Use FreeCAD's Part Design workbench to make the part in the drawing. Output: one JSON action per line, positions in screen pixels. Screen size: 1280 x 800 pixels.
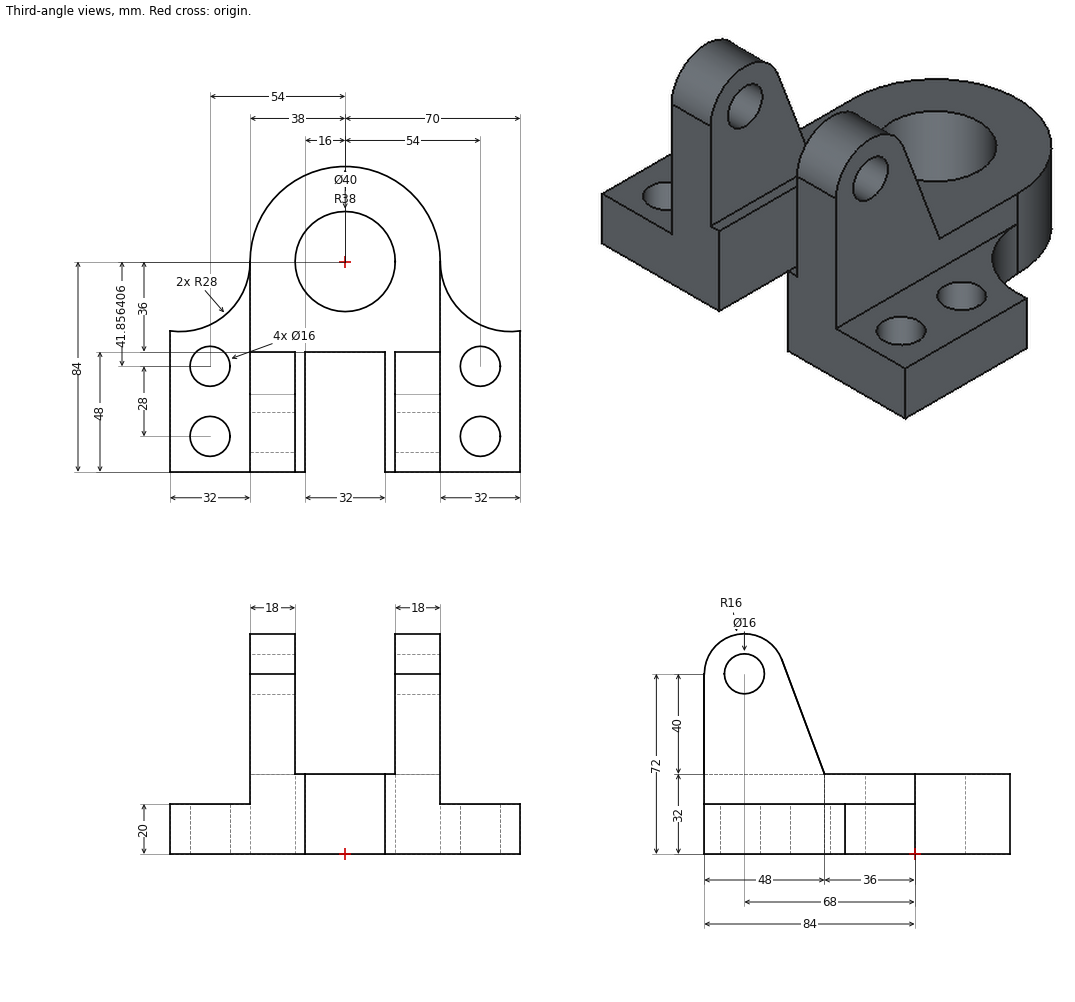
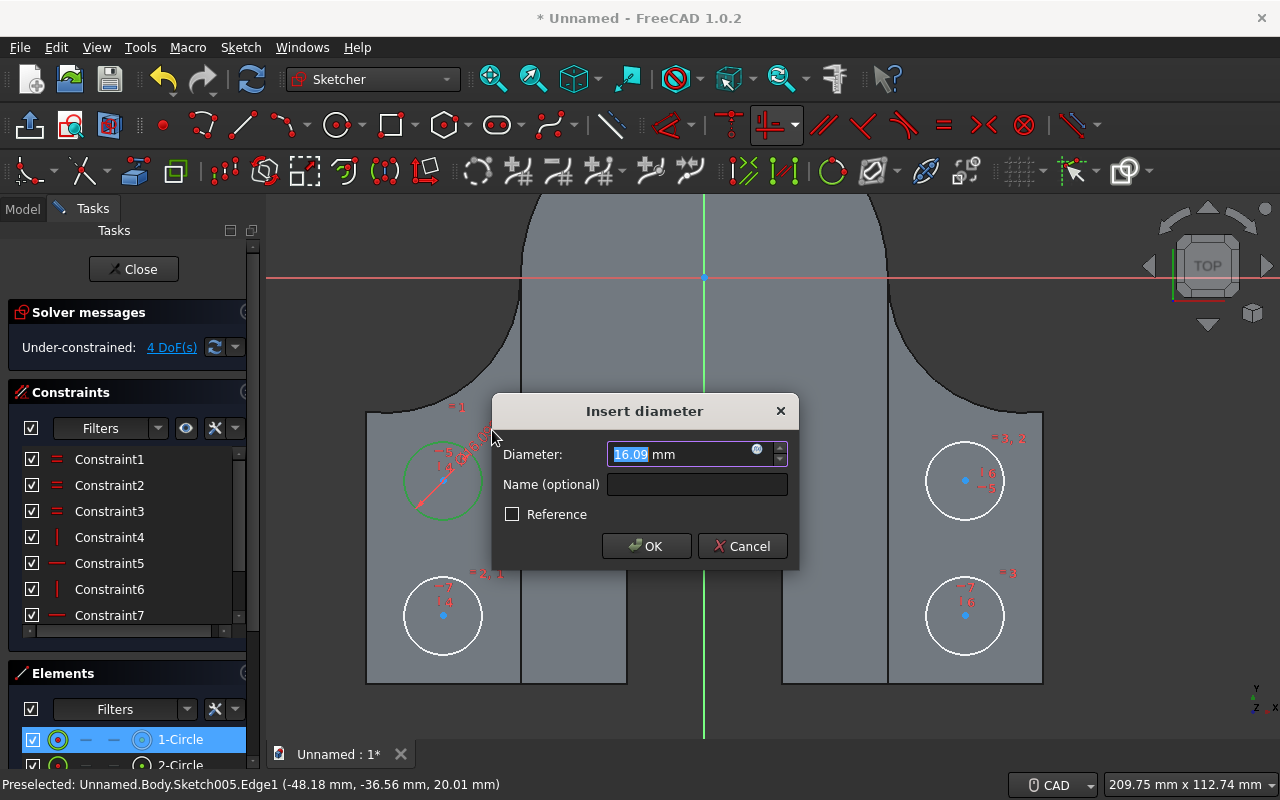
{"action": "type", "text": "16"}
{"action": "key", "text": "Return"}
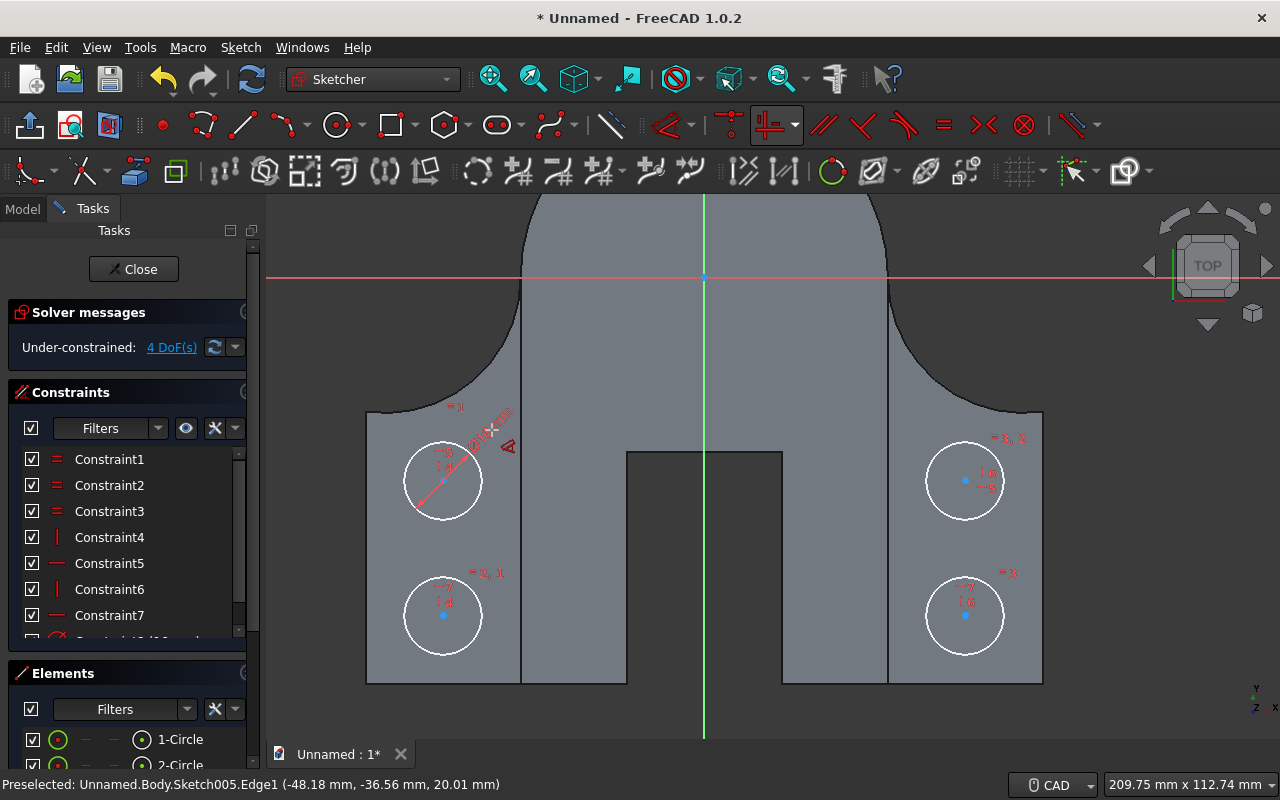
{"action": "left_click", "coordinate": [443, 481]}
{"action": "left_click", "coordinate": [574, 244]}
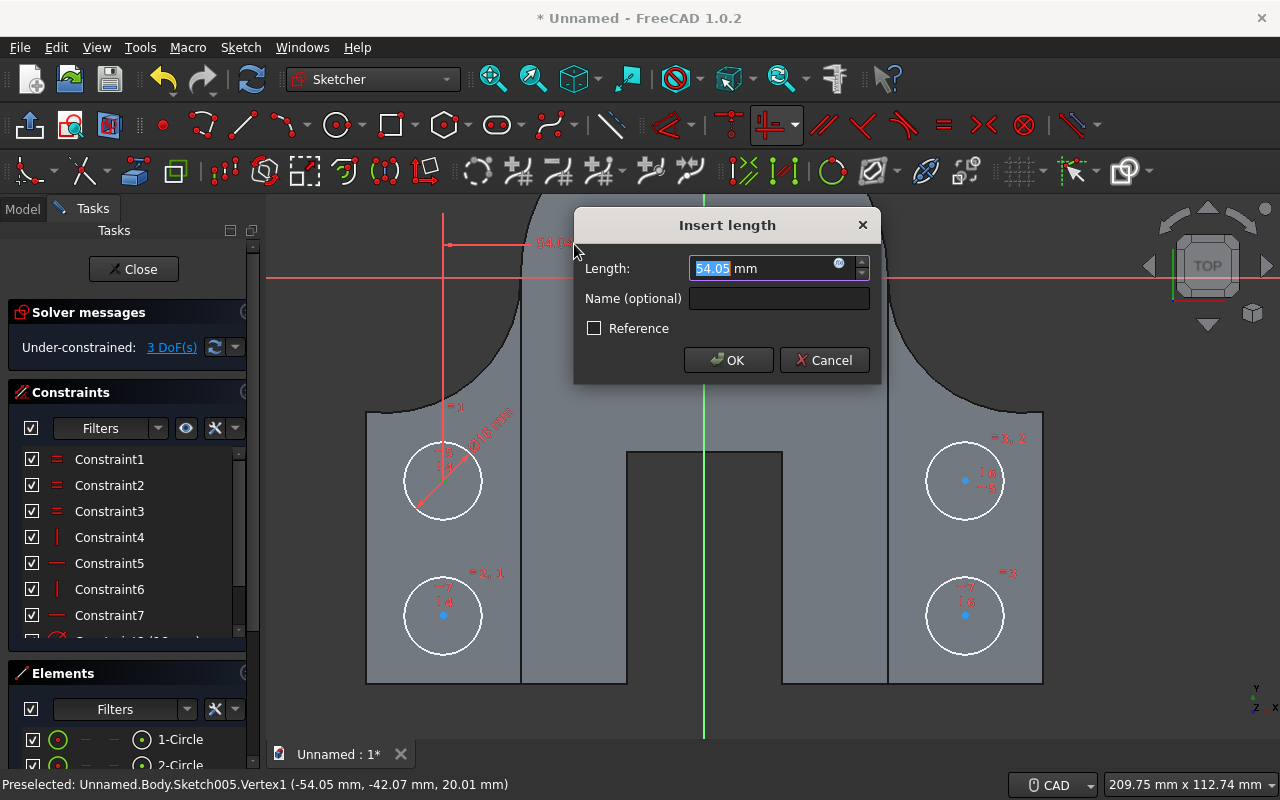
{"action": "type", "text": "54"}
{"action": "key", "text": "Return"}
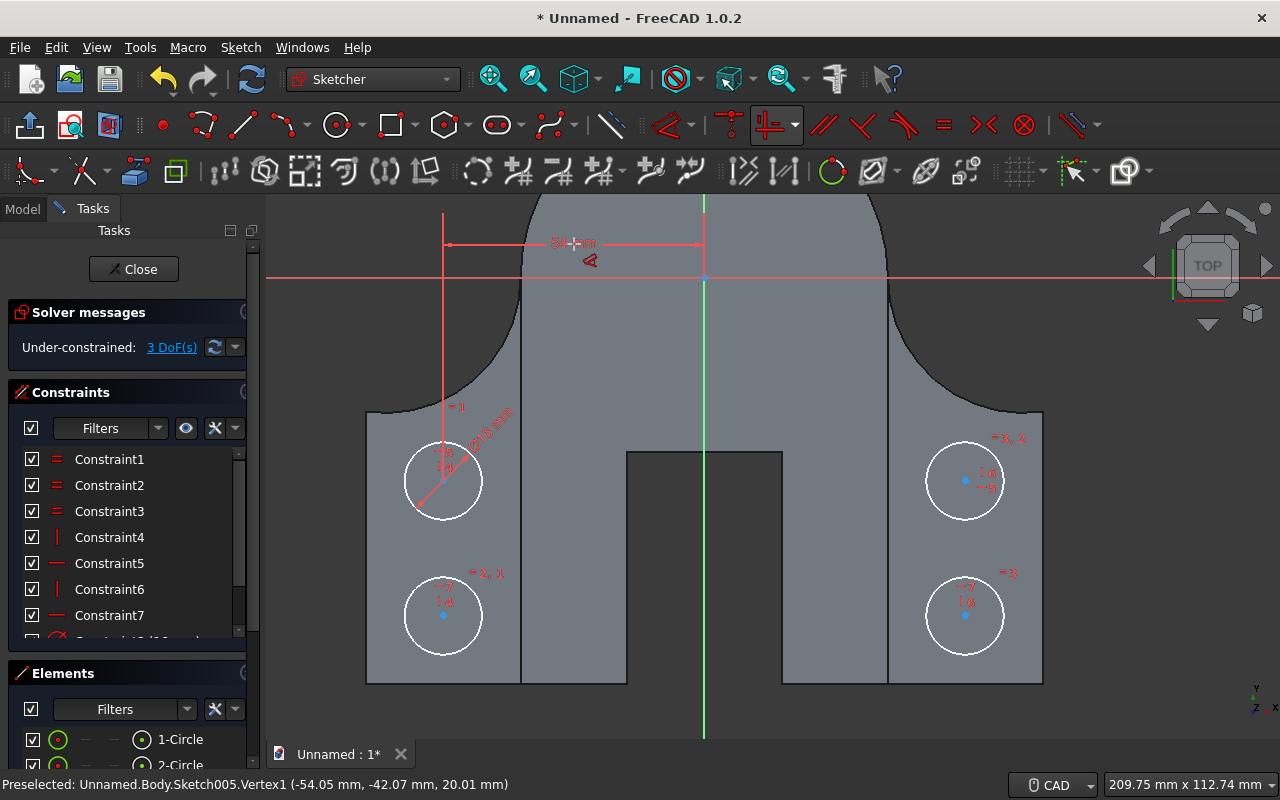
{"action": "left_click", "coordinate": [965, 481]}
{"action": "left_click", "coordinate": [835, 244]}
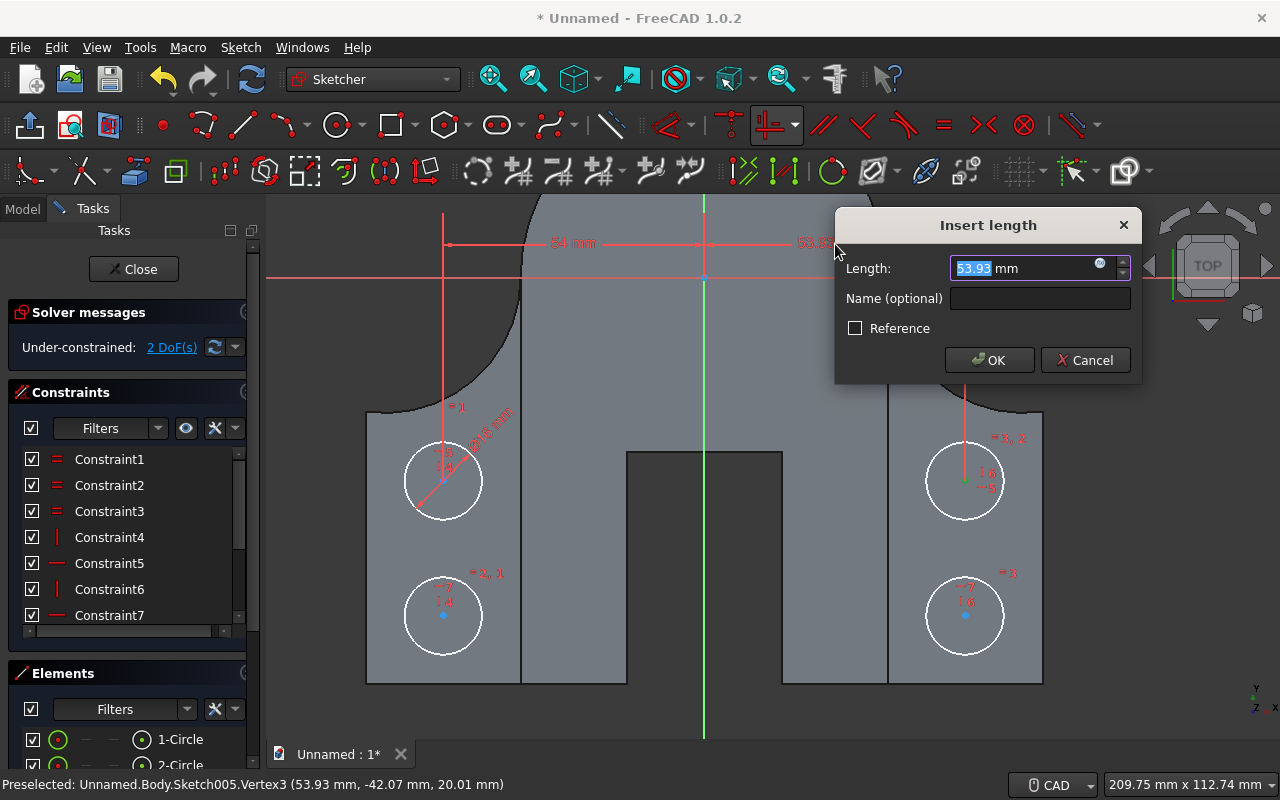
{"action": "type", "text": "54"}
{"action": "key", "text": "Return"}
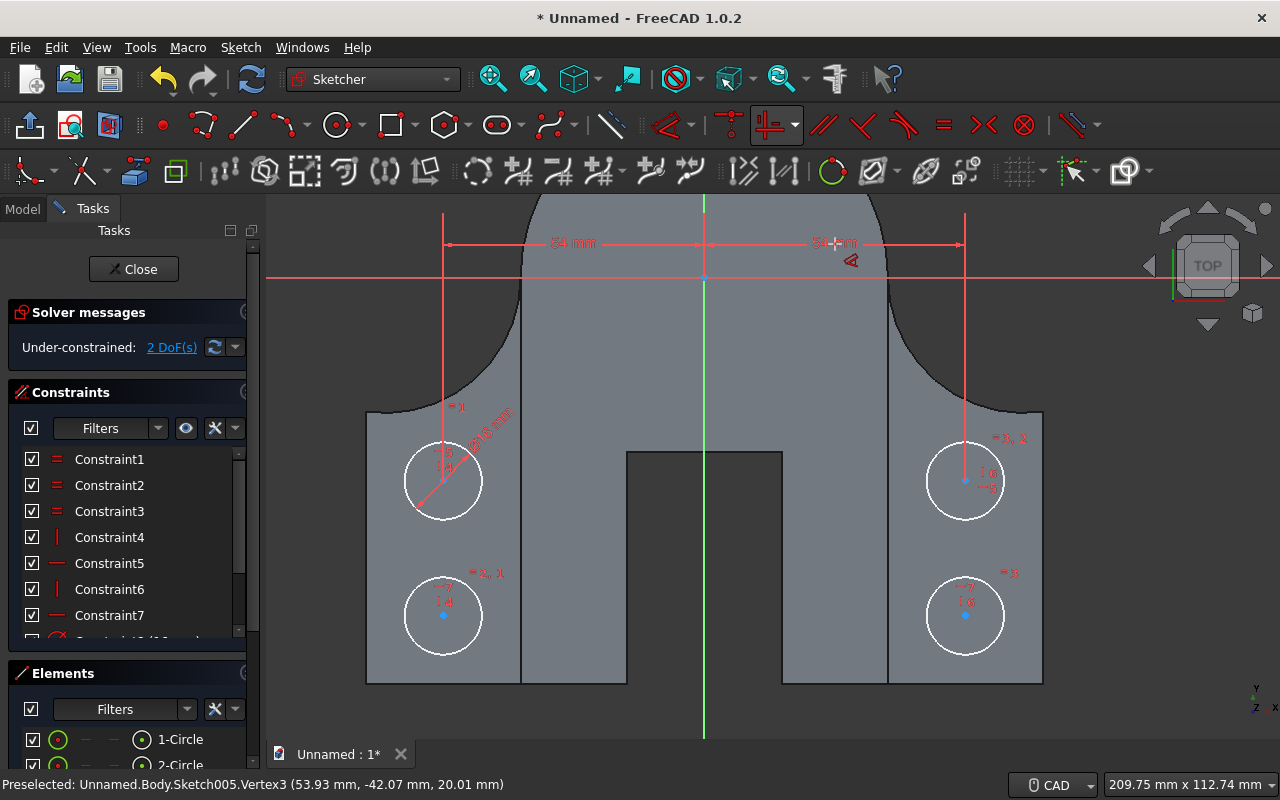
{"action": "left_click", "coordinate": [443, 481]}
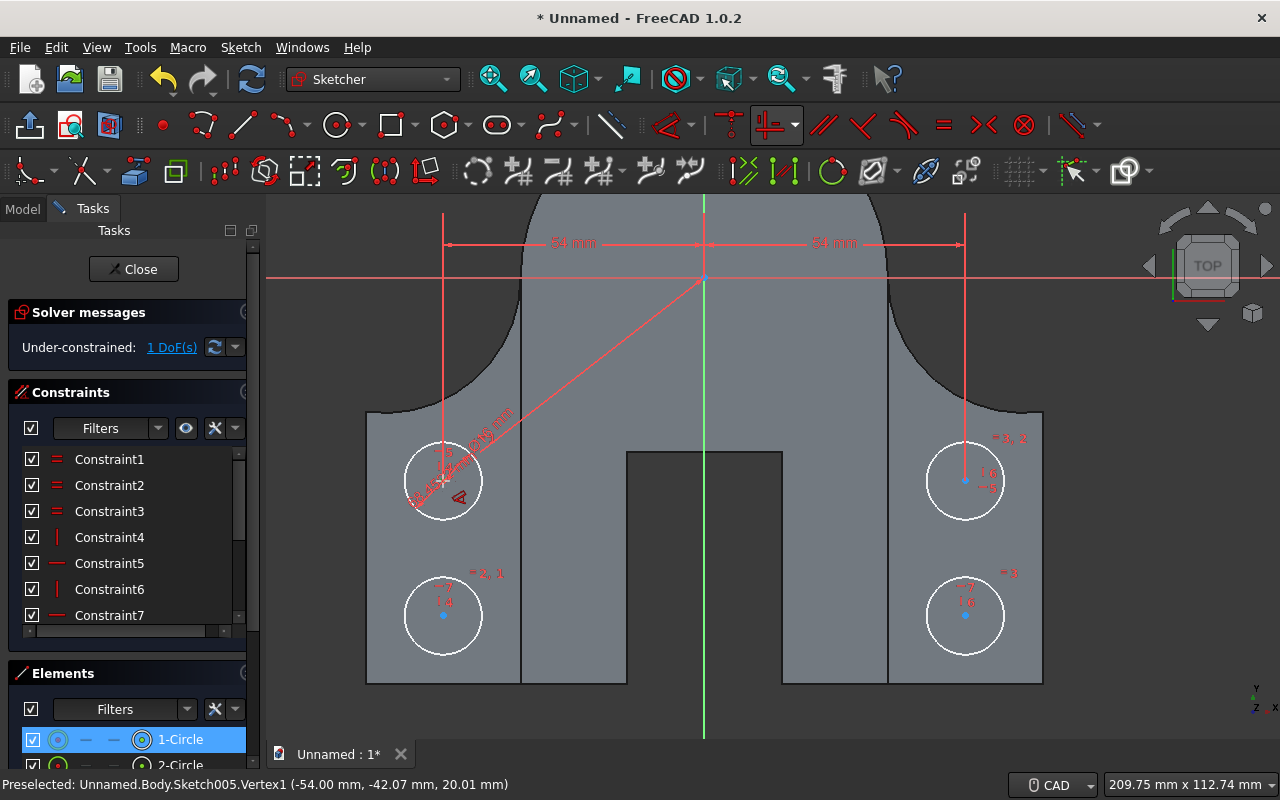
{"action": "left_click", "coordinate": [443, 616]}
{"action": "left_click", "coordinate": [409, 549]}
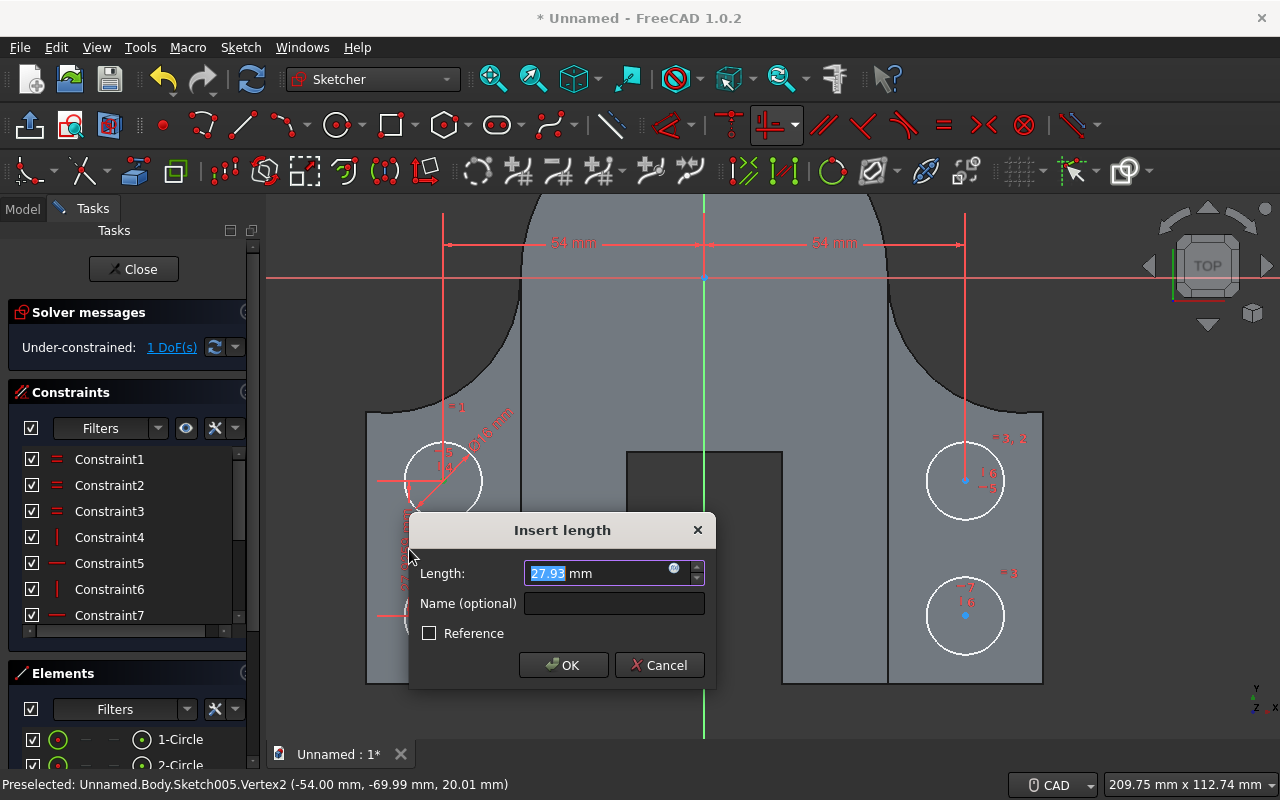
{"action": "type", "text": "28"}
{"action": "key", "text": "Return"}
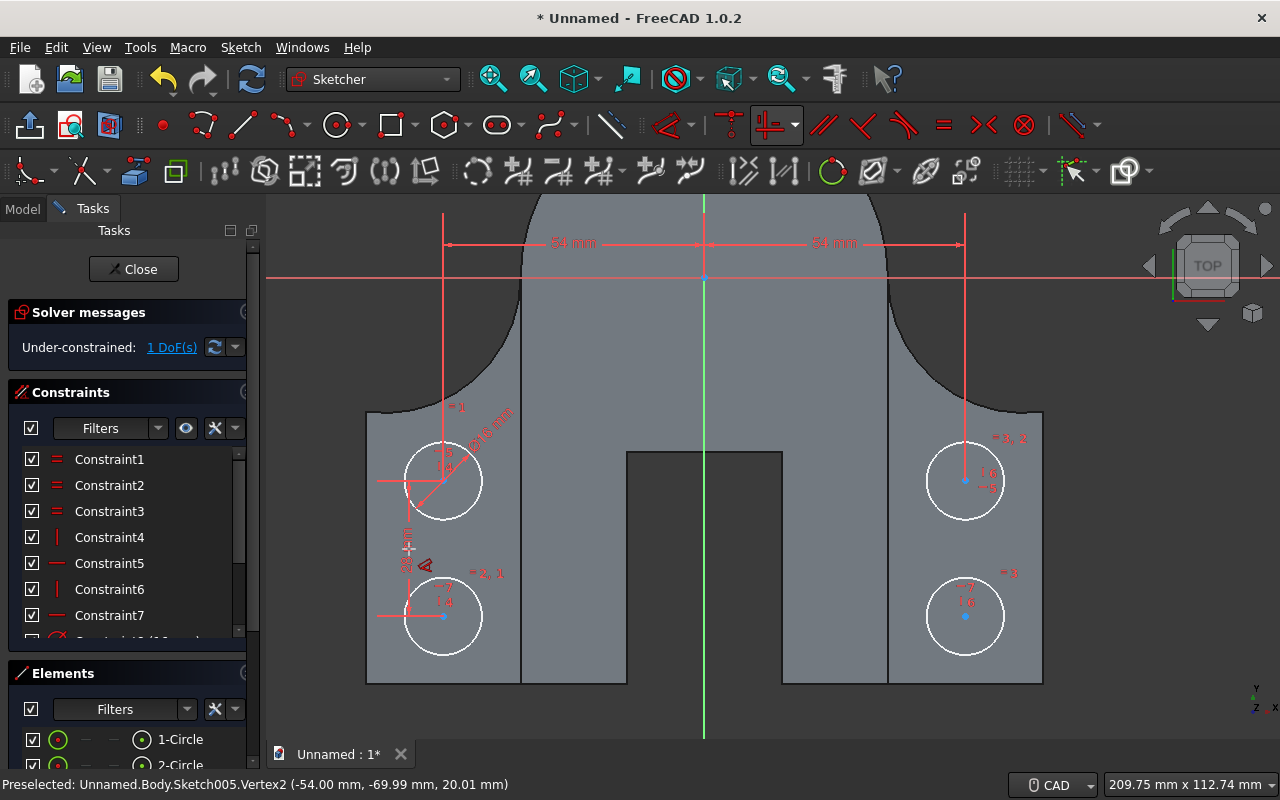
{"action": "left_click", "coordinate": [443, 481]}
{"action": "left_click", "coordinate": [409, 379]}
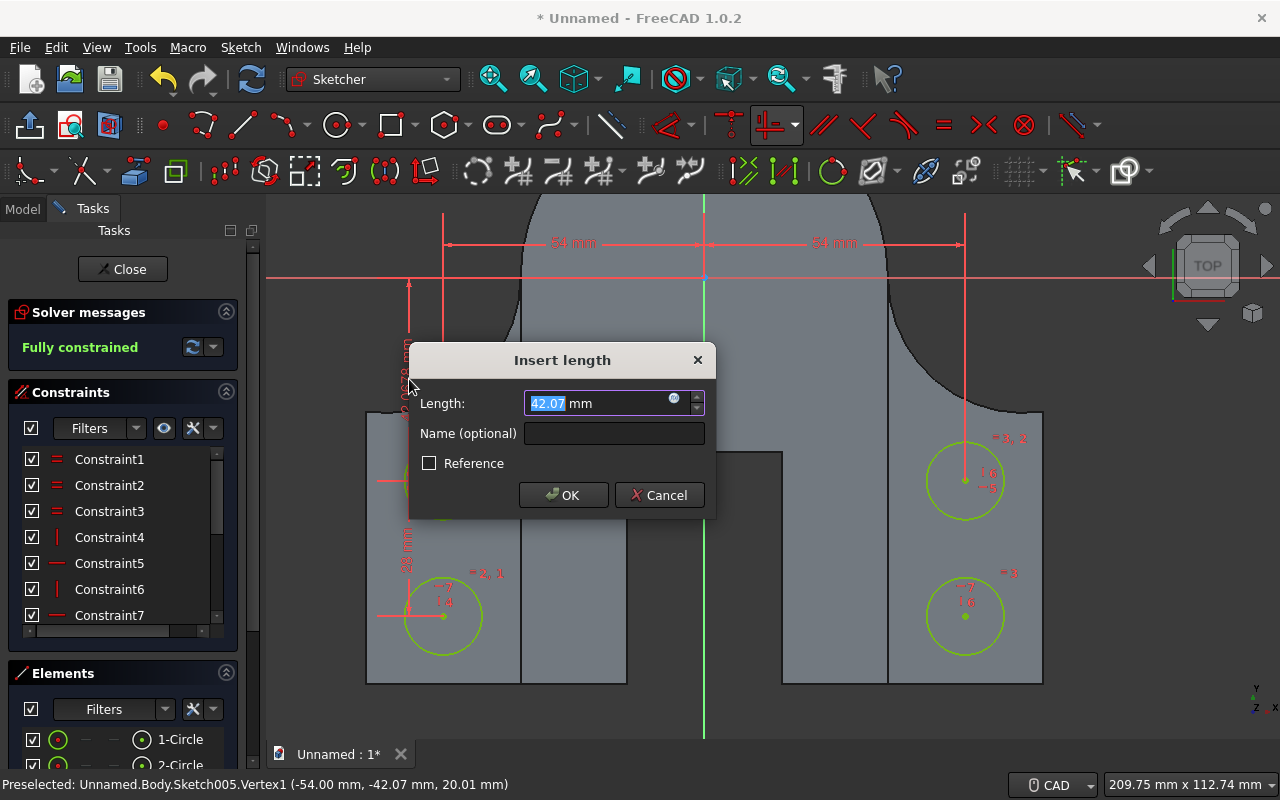
{"action": "type", "text": "41.856406"}
{"action": "key", "text": "Return"}
{"action": "key", "text": "Escape"}